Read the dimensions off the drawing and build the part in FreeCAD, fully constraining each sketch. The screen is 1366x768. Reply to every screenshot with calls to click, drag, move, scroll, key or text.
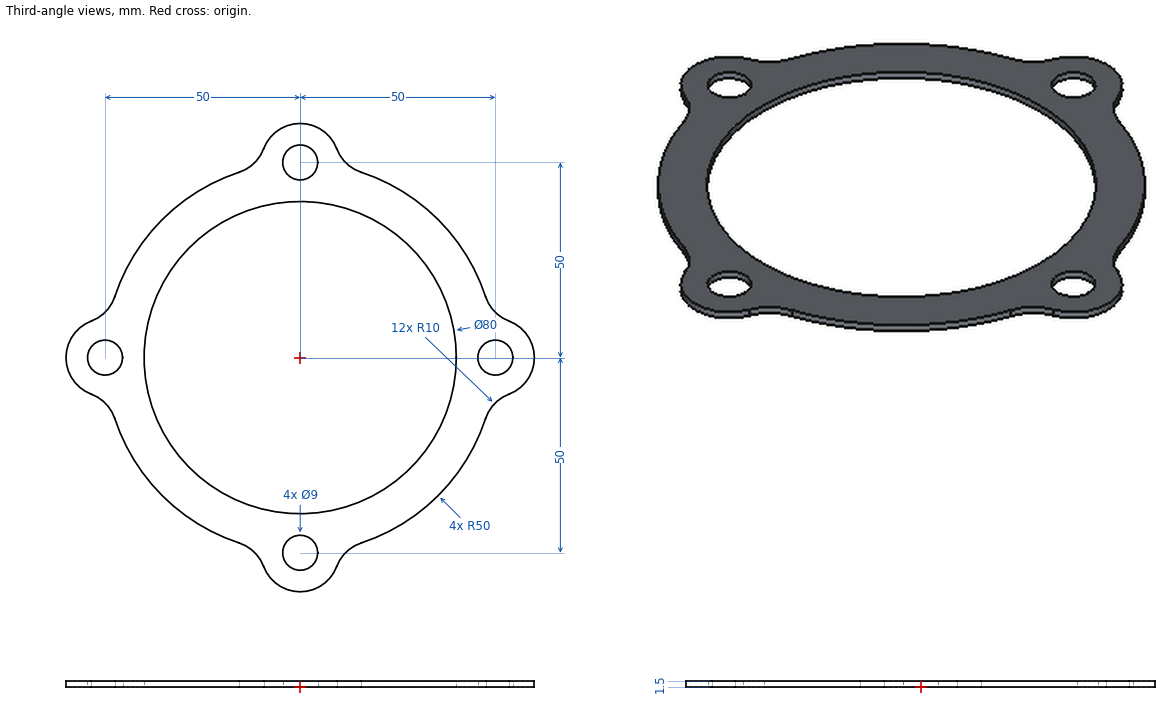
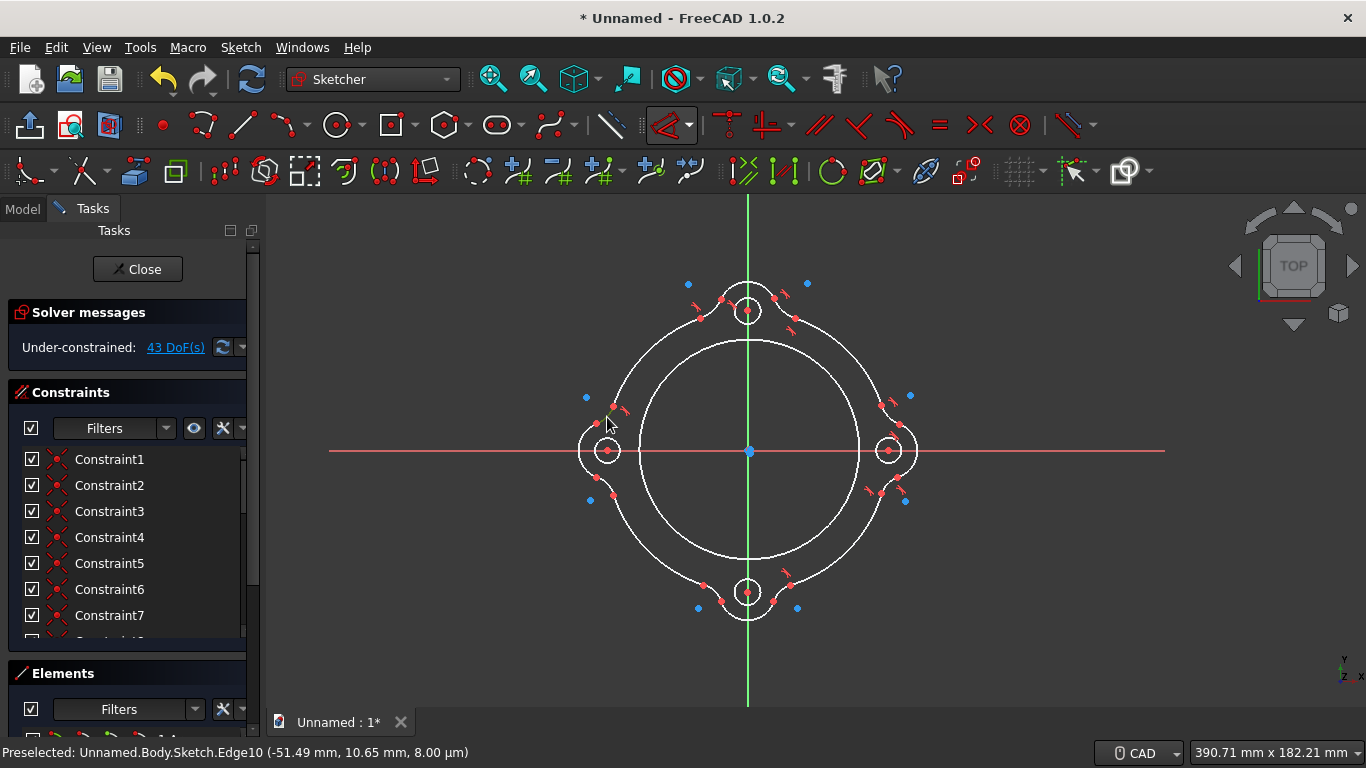
click(582, 437)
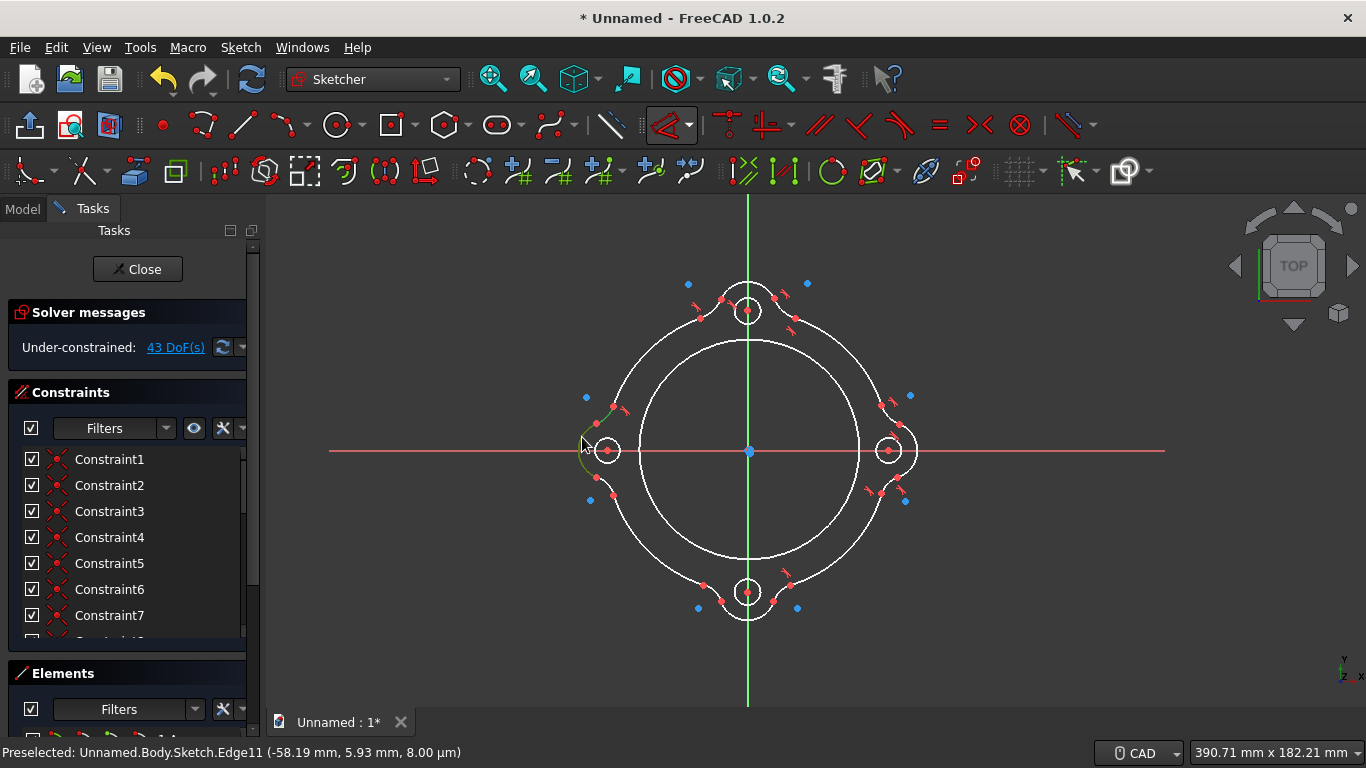
click(900, 126)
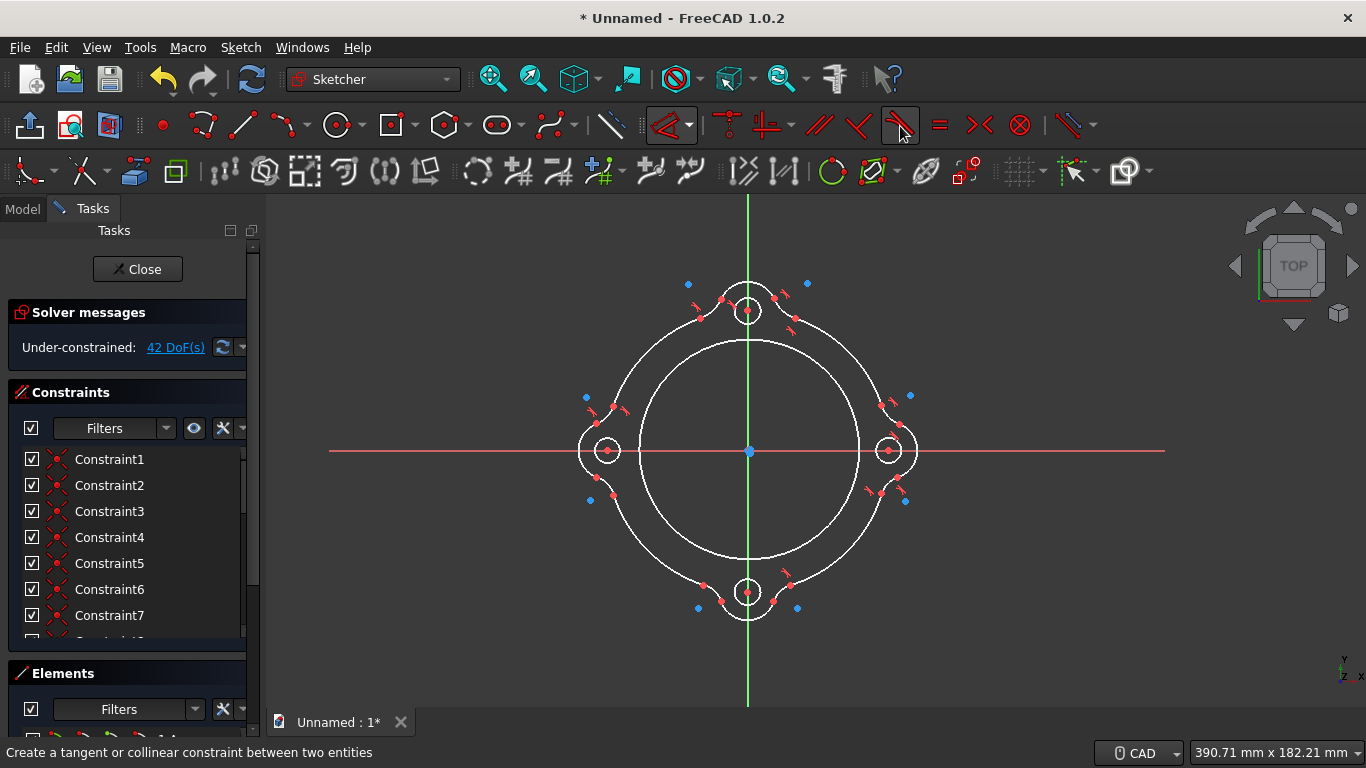
click(582, 437)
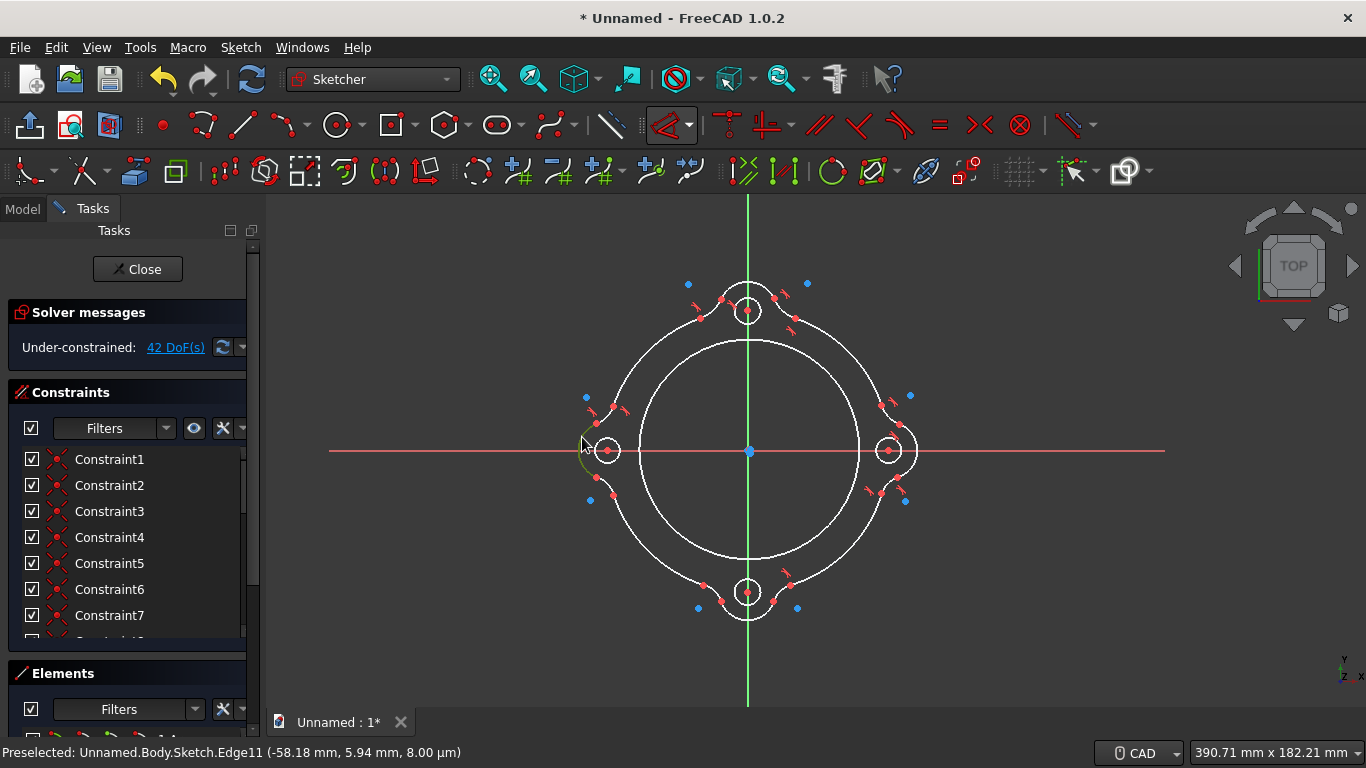
click(608, 484)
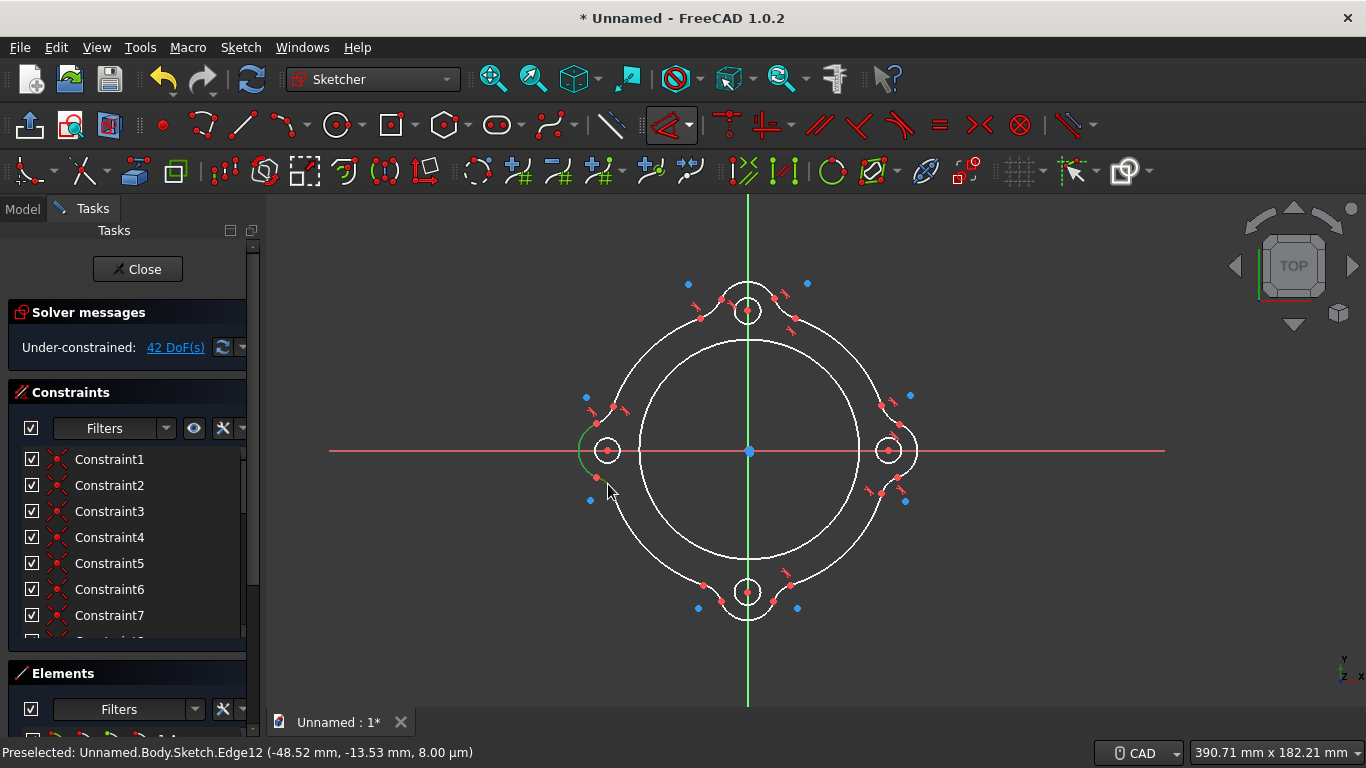
click(900, 126)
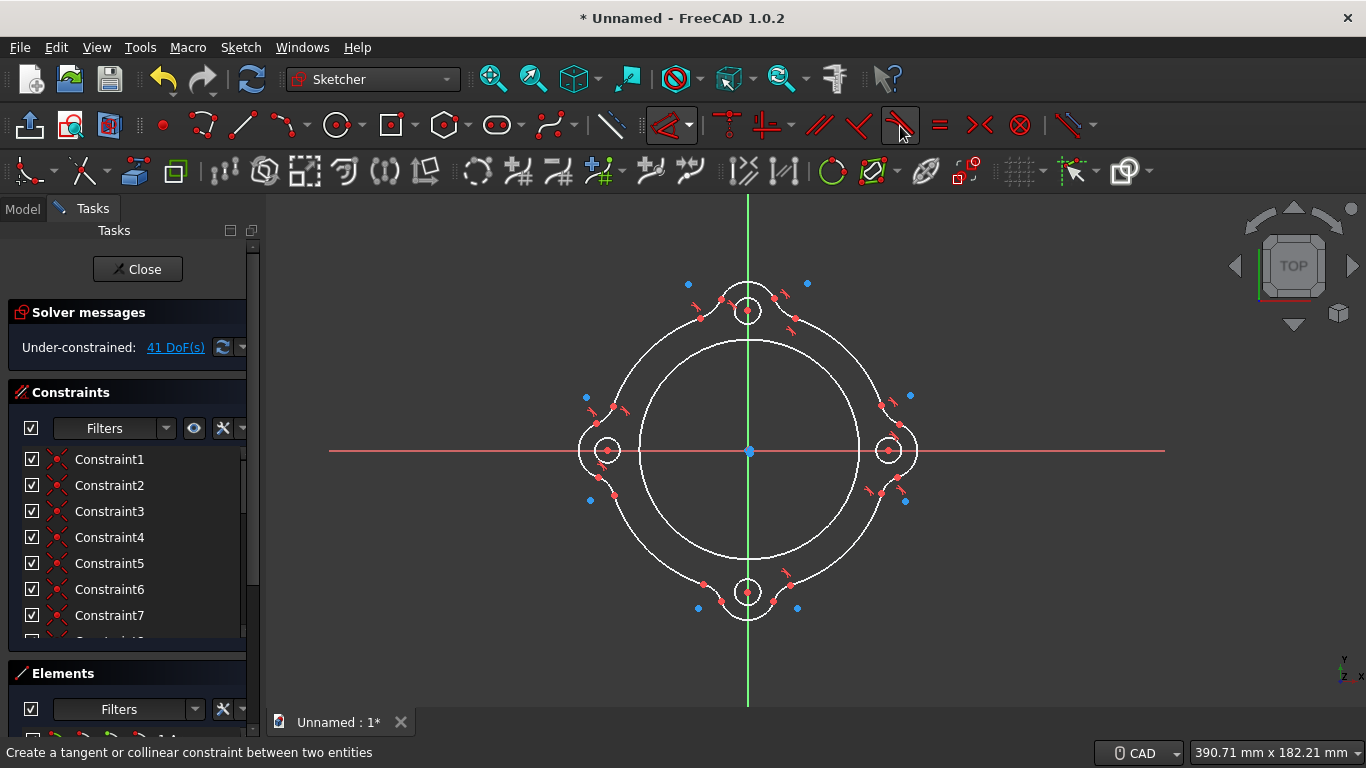
click(609, 484)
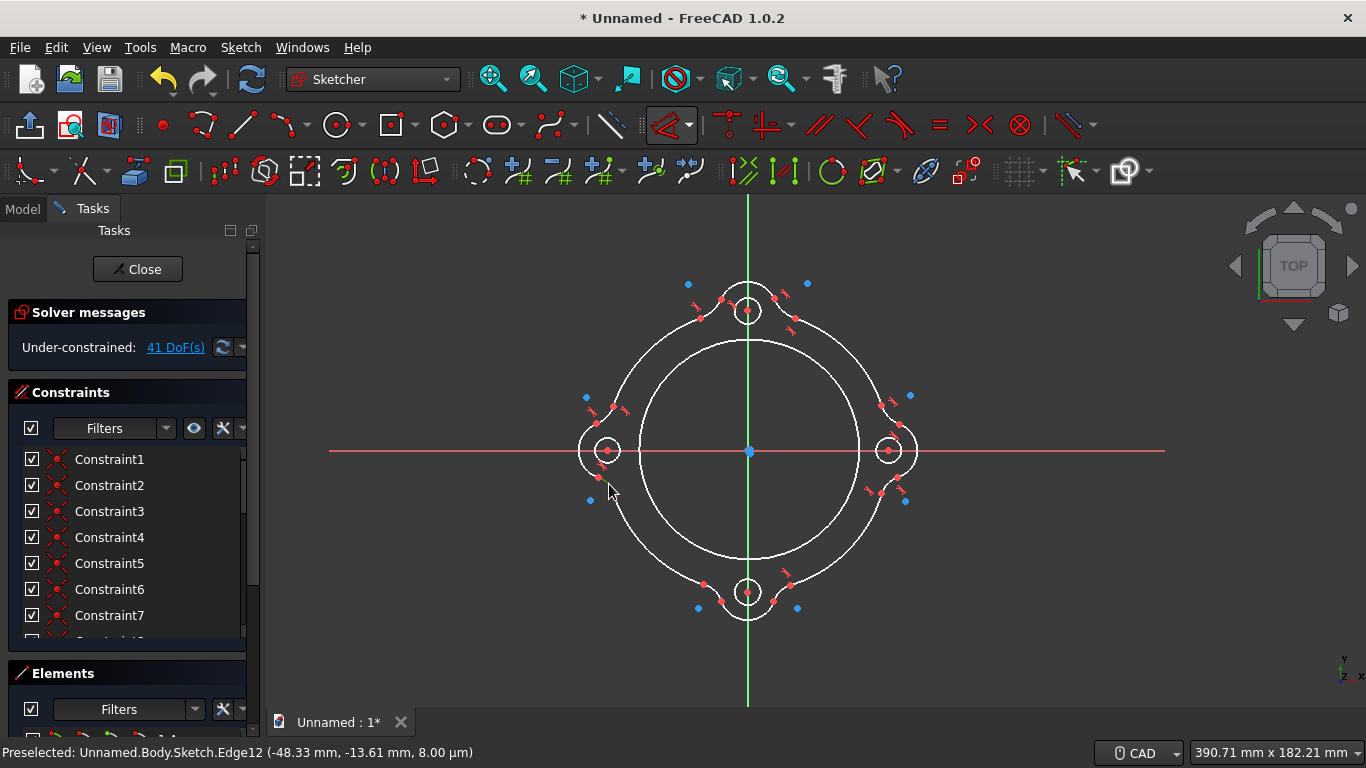
click(632, 530)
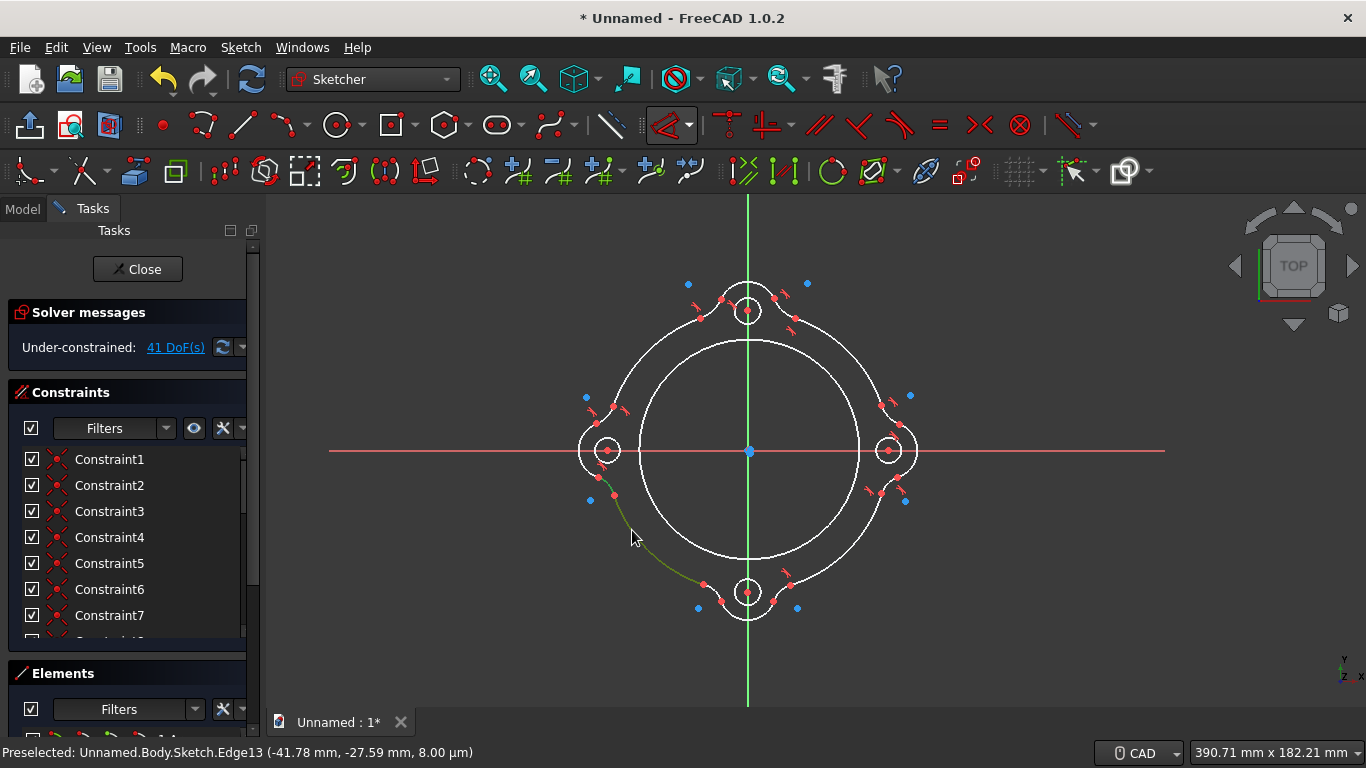
click(900, 126)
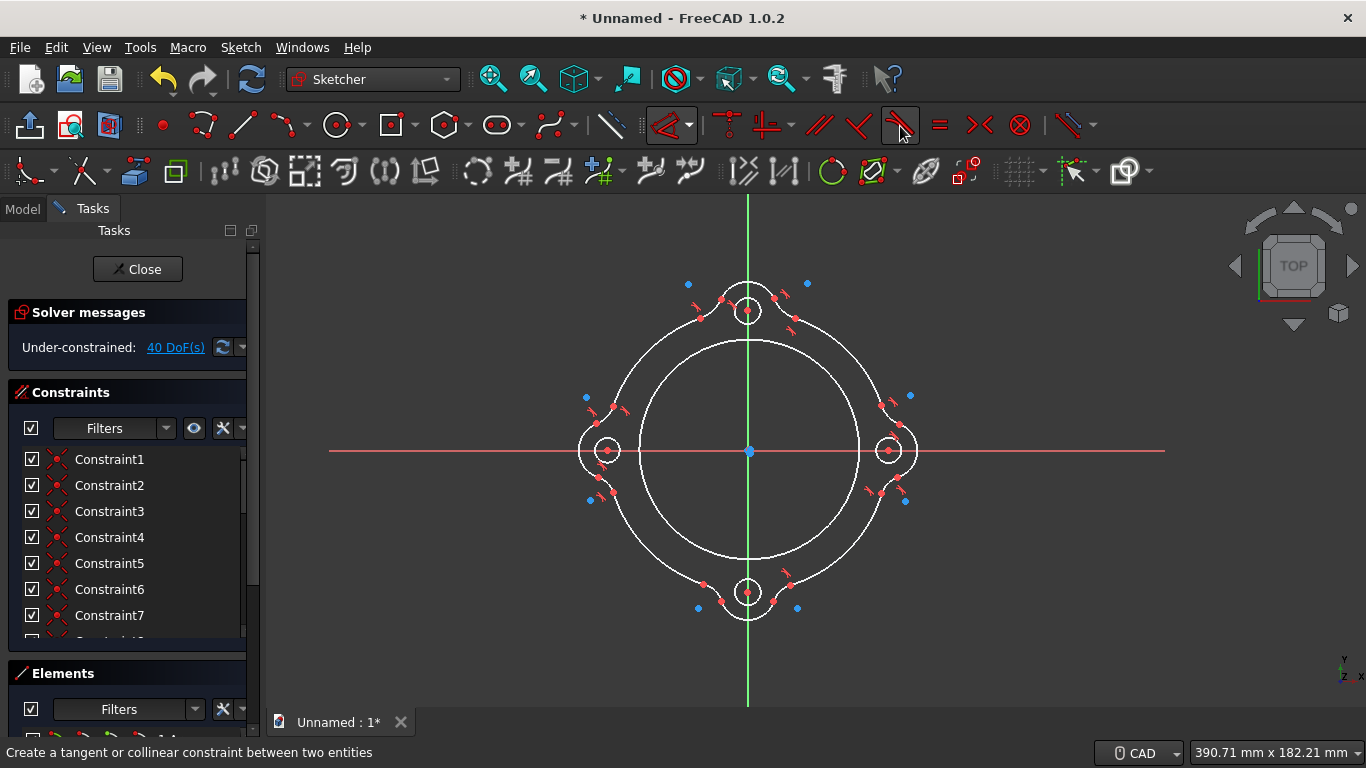
click(631, 529)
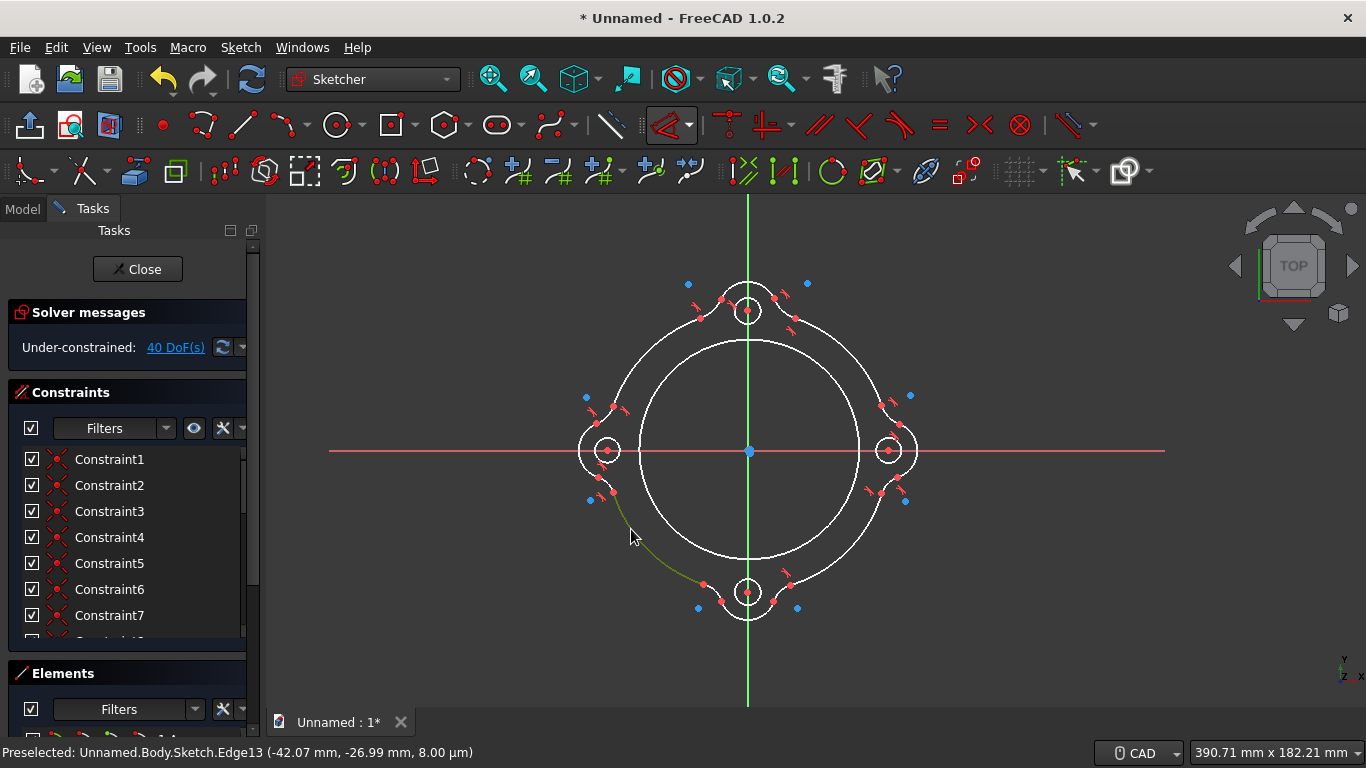
click(715, 591)